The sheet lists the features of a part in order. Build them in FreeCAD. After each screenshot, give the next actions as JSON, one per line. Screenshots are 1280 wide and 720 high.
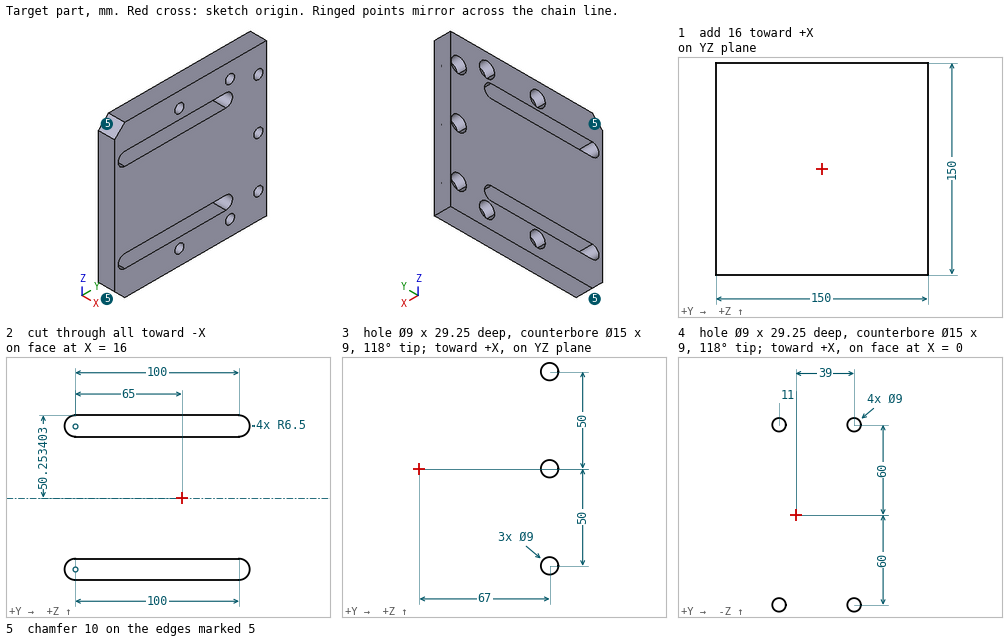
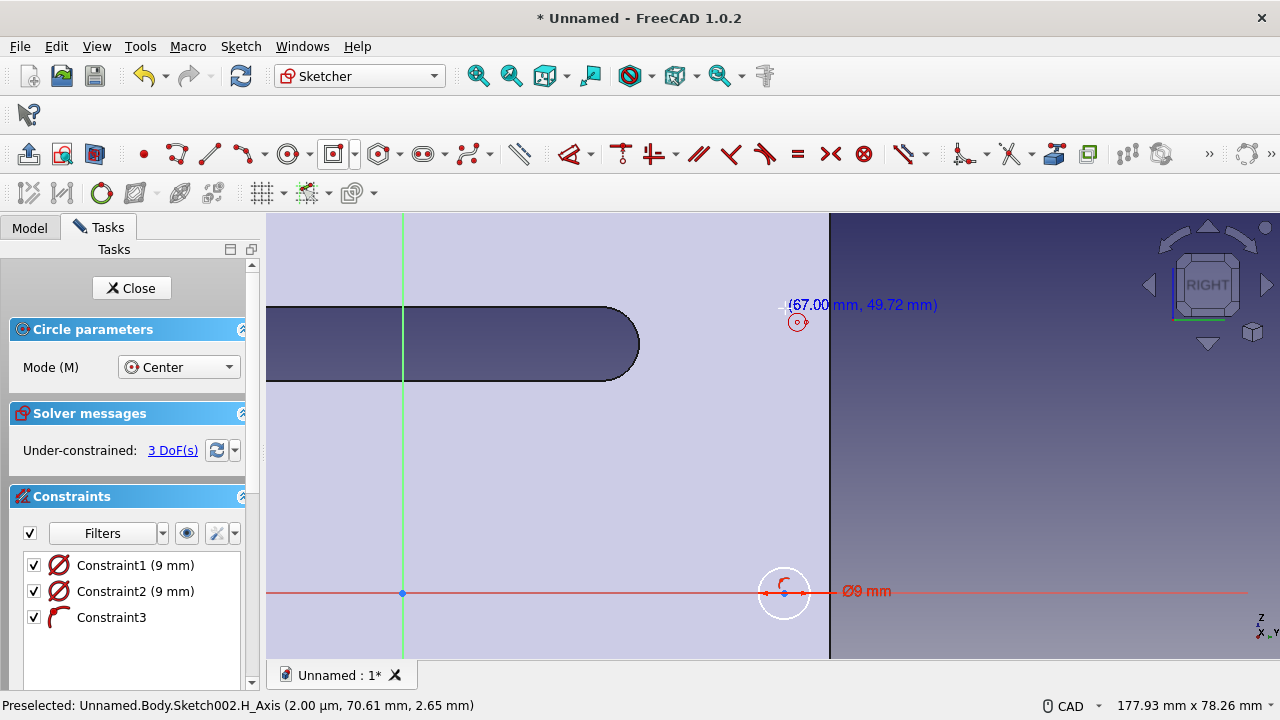
{"action": "left_click", "coordinate": [784, 308]}
{"action": "mouse_move", "coordinate": [802, 290]}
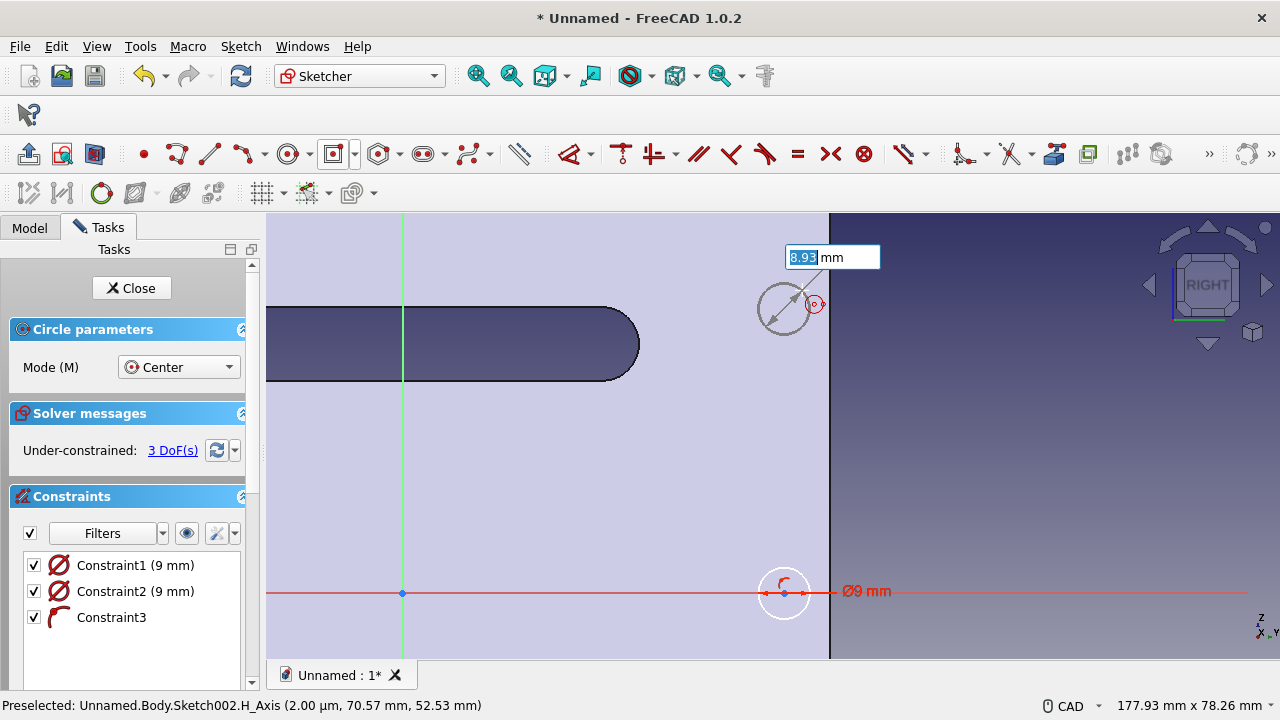
{"action": "type", "text": "9"}
{"action": "key", "text": "Return"}
{"action": "key", "text": "Escape"}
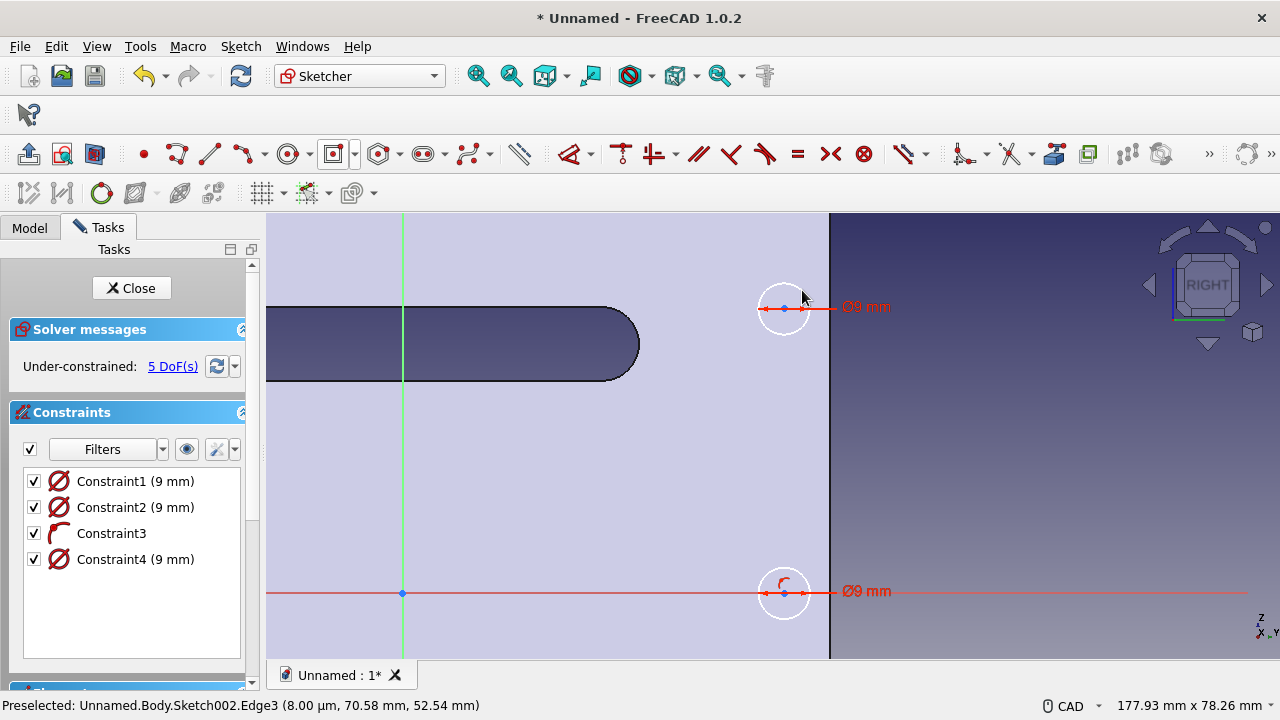
{"action": "scroll", "coordinate": [785, 308], "scroll_direction": "down", "scroll_amount": 4}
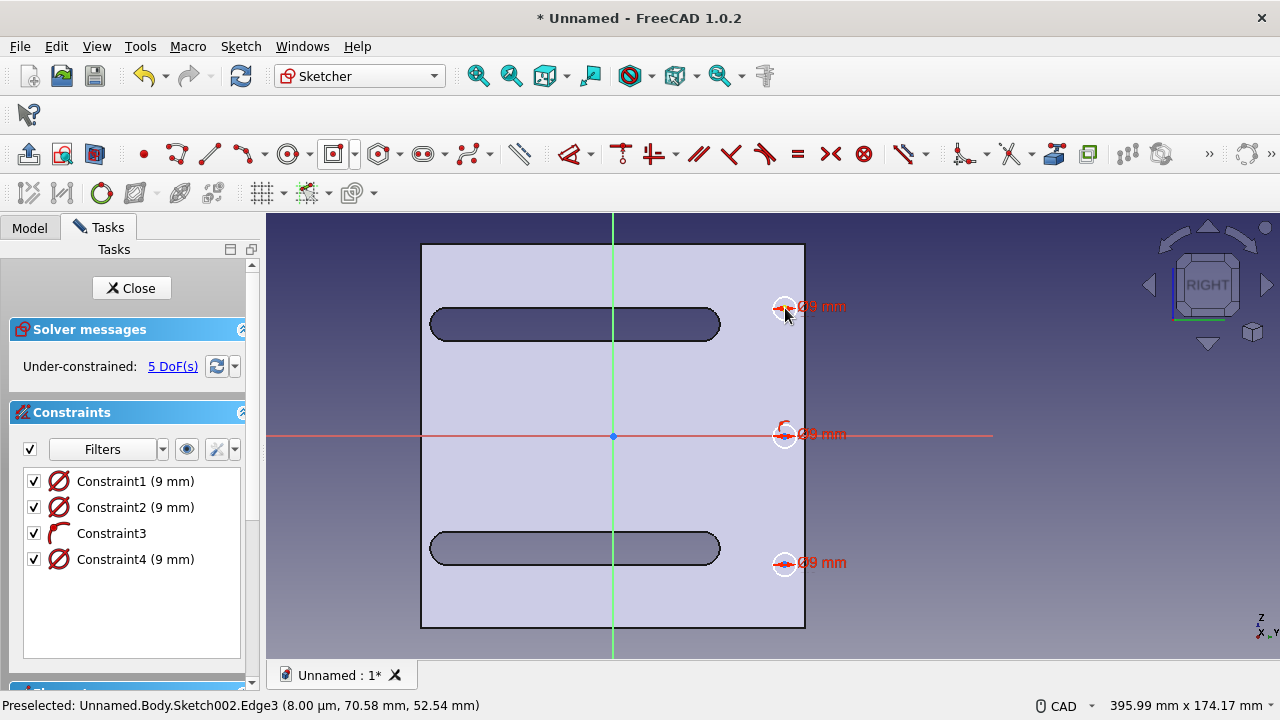
{"action": "left_click", "coordinate": [785, 565]}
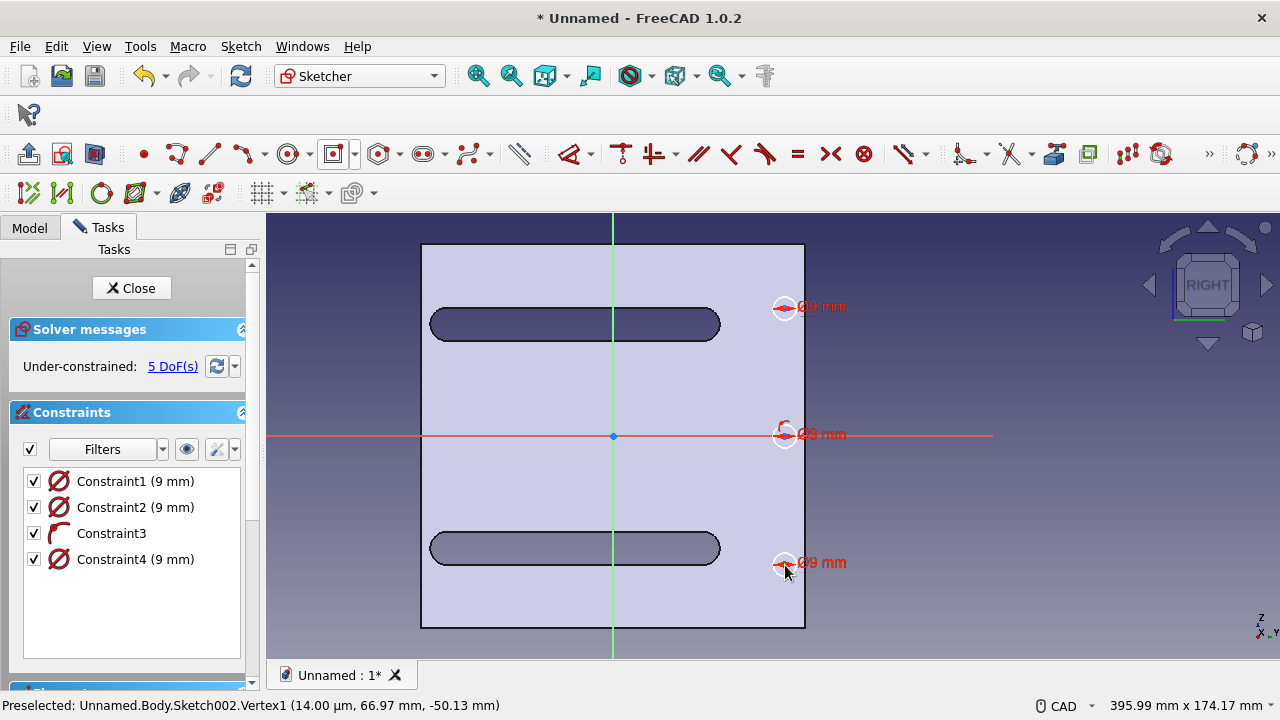
{"action": "left_click", "coordinate": [785, 436]}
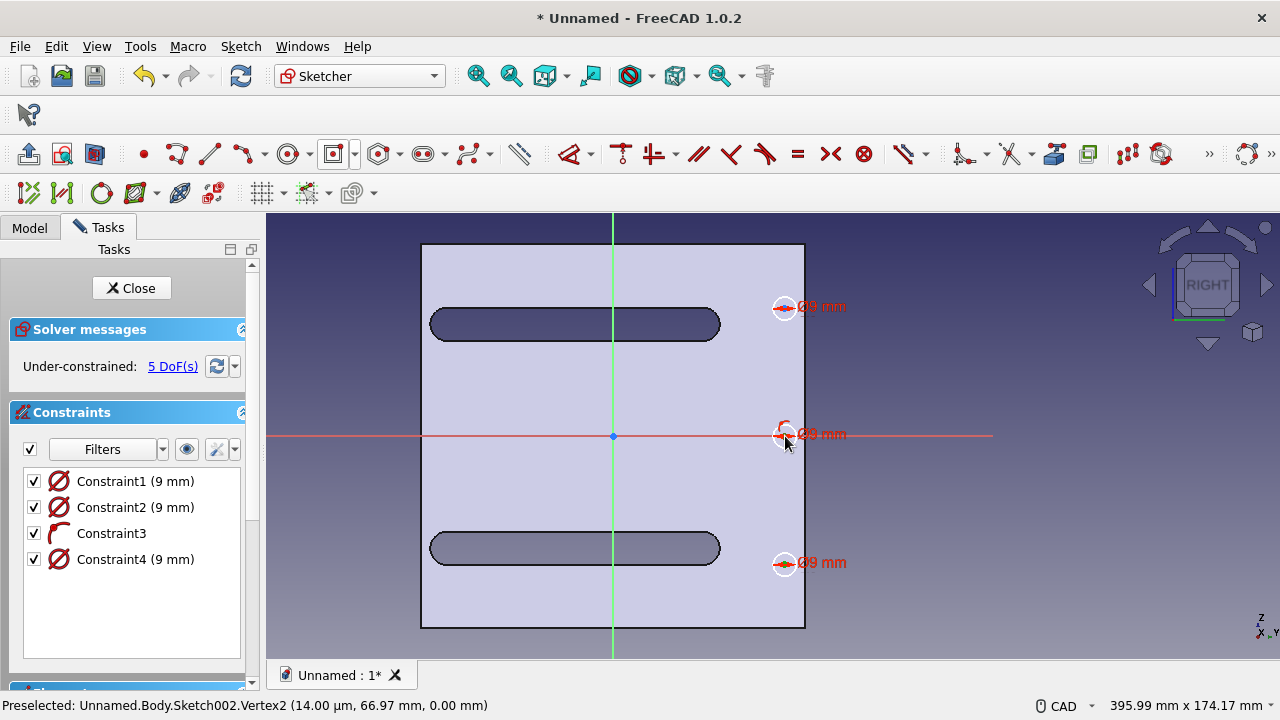
{"action": "left_click", "coordinate": [676, 154]}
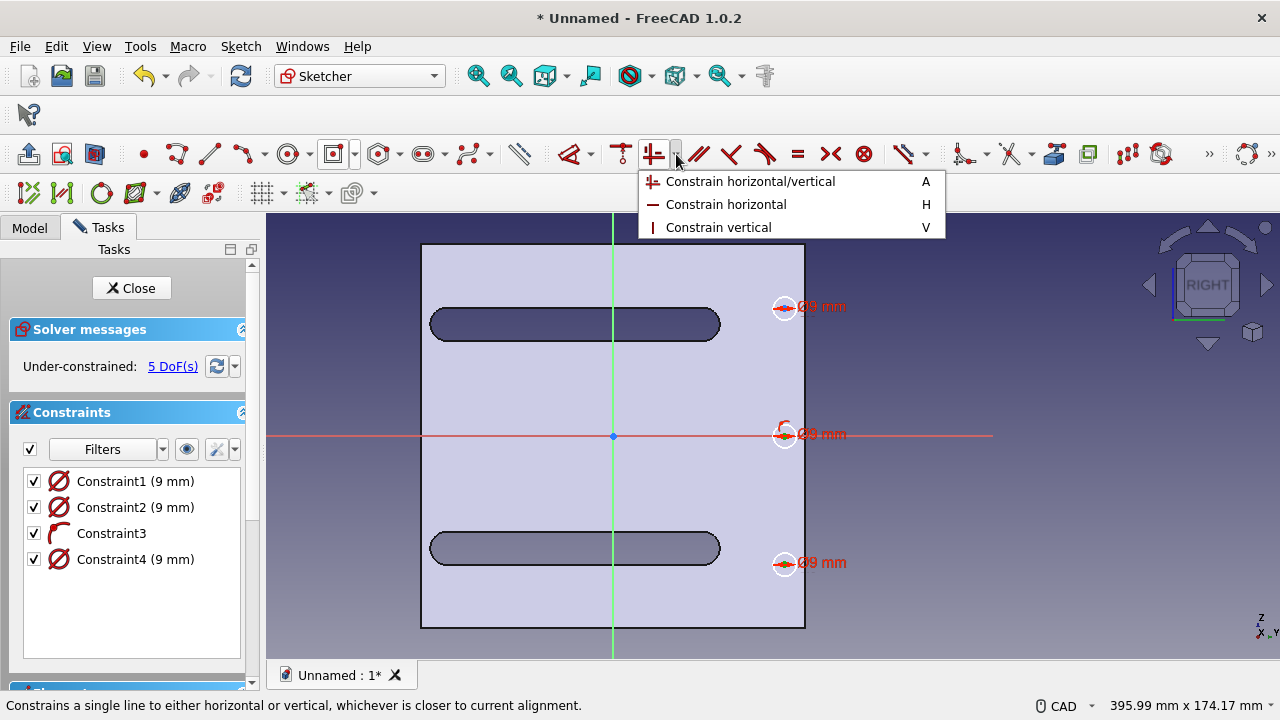
{"action": "left_click", "coordinate": [792, 228]}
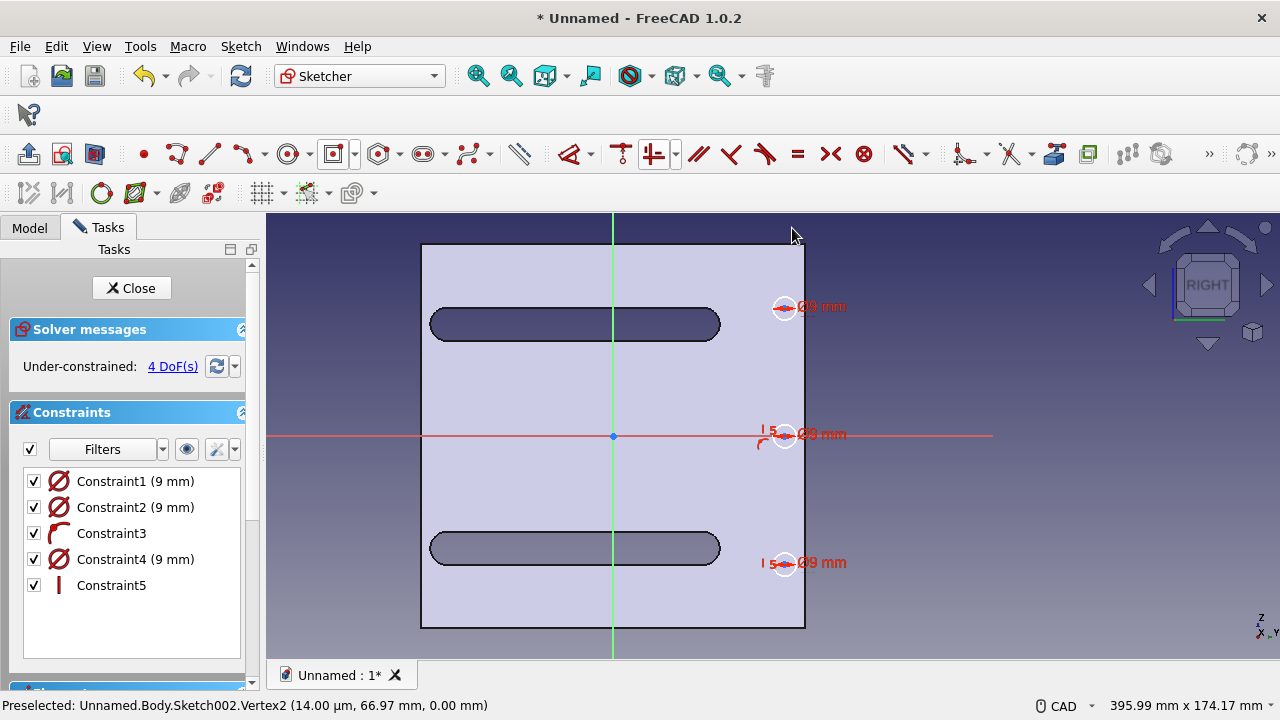
{"action": "left_click", "coordinate": [785, 436]}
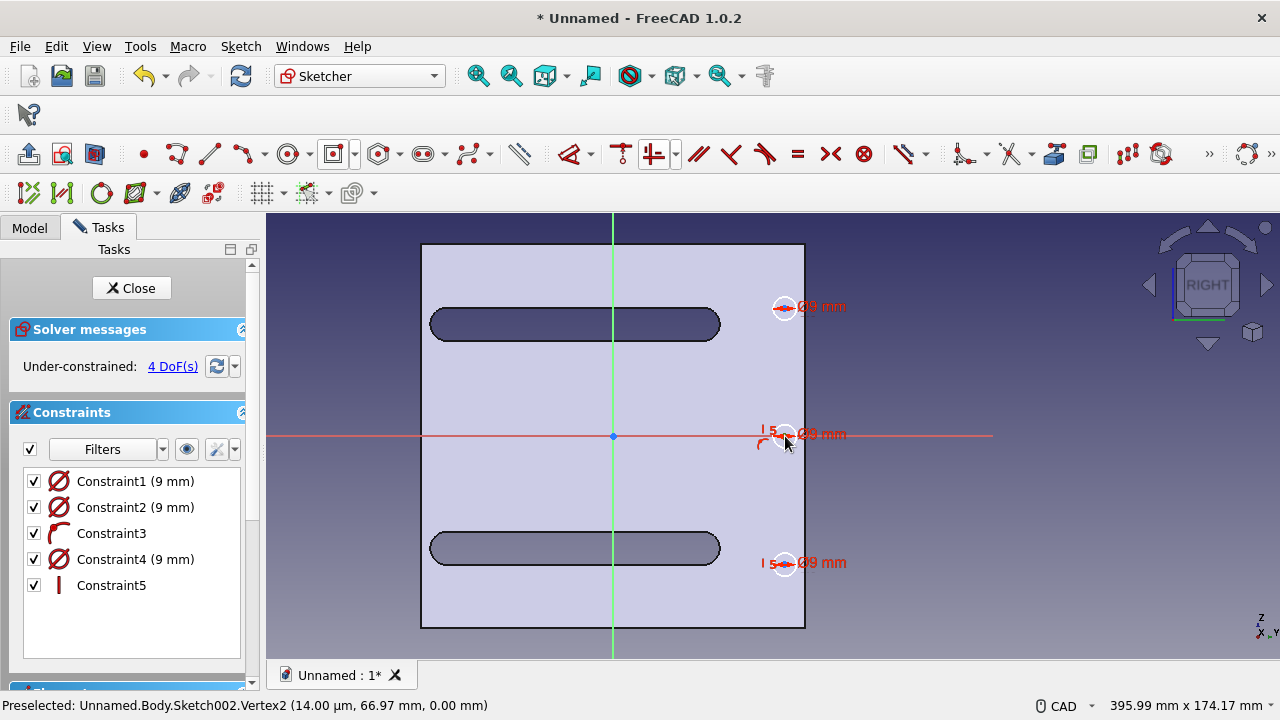
{"action": "left_click", "coordinate": [785, 309]}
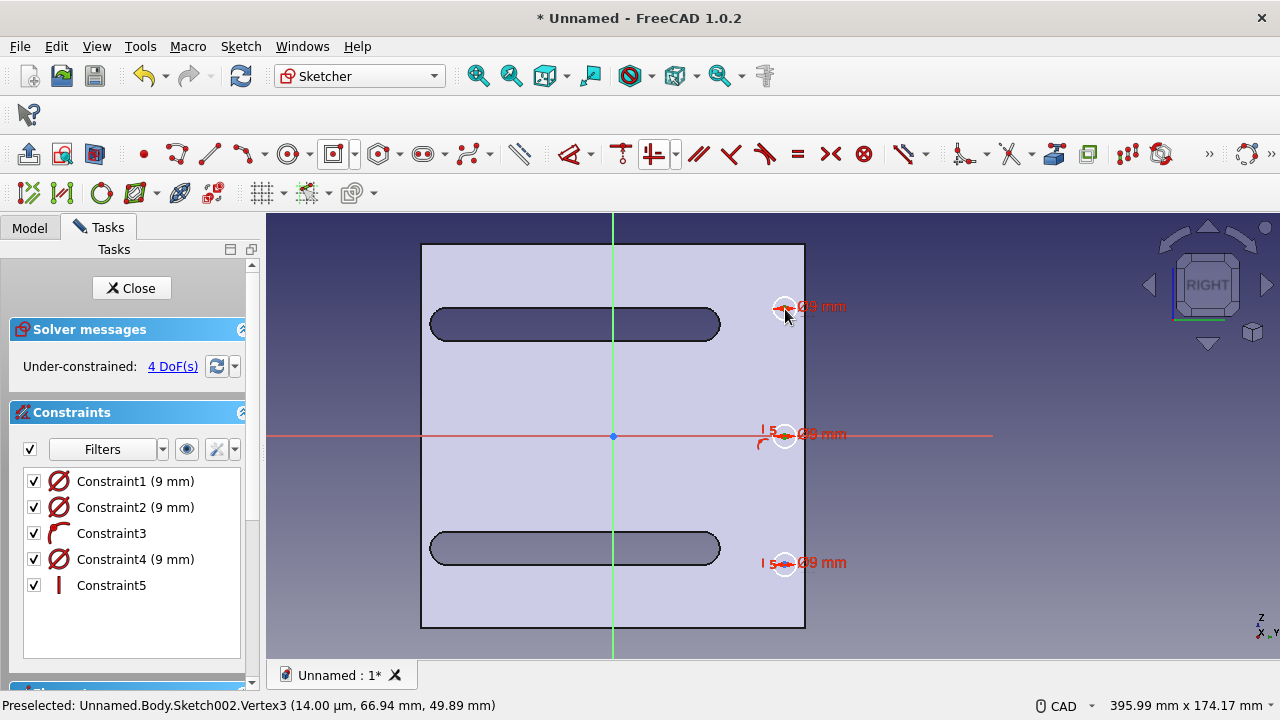
{"action": "left_click", "coordinate": [676, 154]}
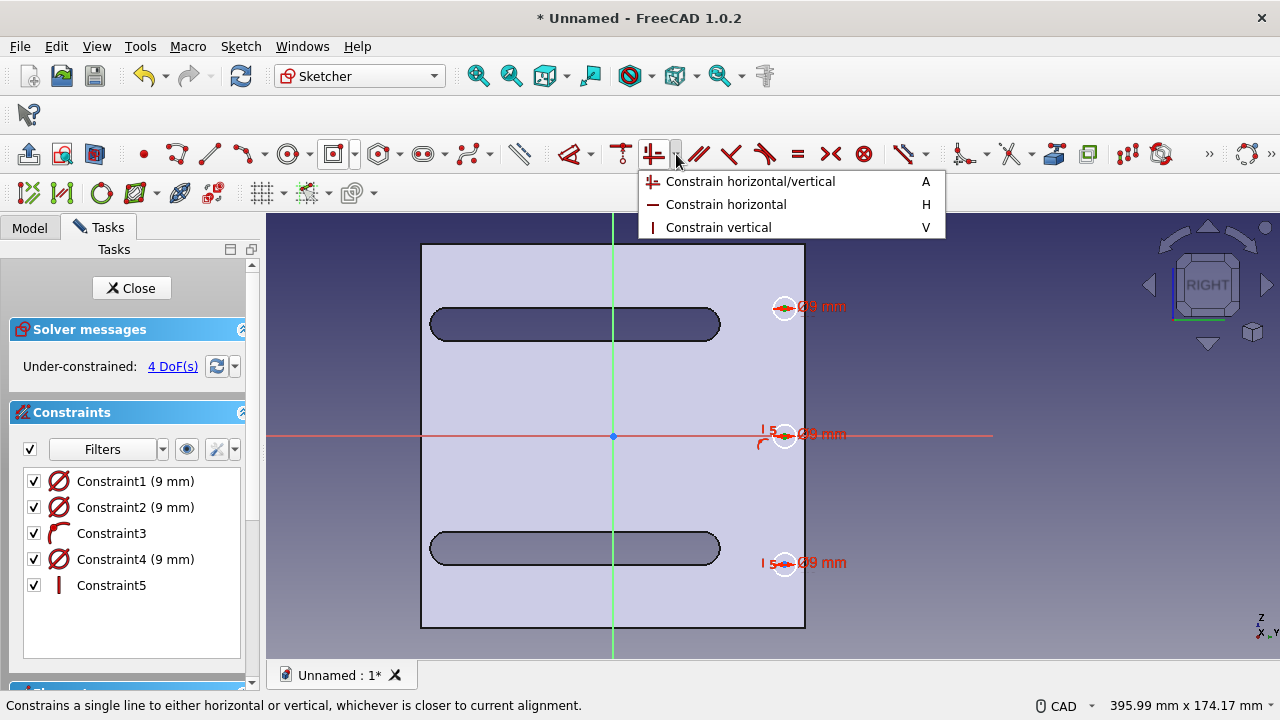
{"action": "left_click", "coordinate": [792, 228]}